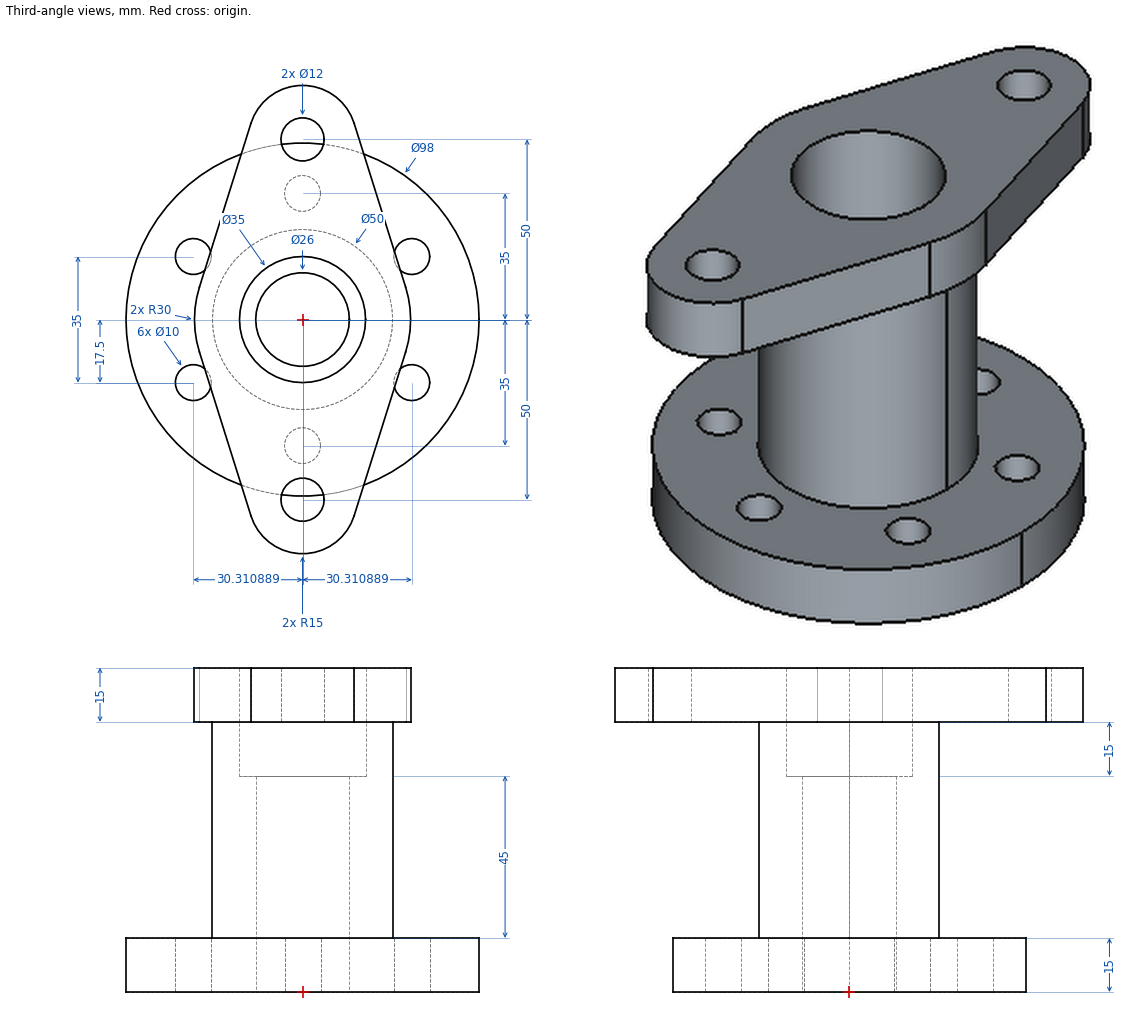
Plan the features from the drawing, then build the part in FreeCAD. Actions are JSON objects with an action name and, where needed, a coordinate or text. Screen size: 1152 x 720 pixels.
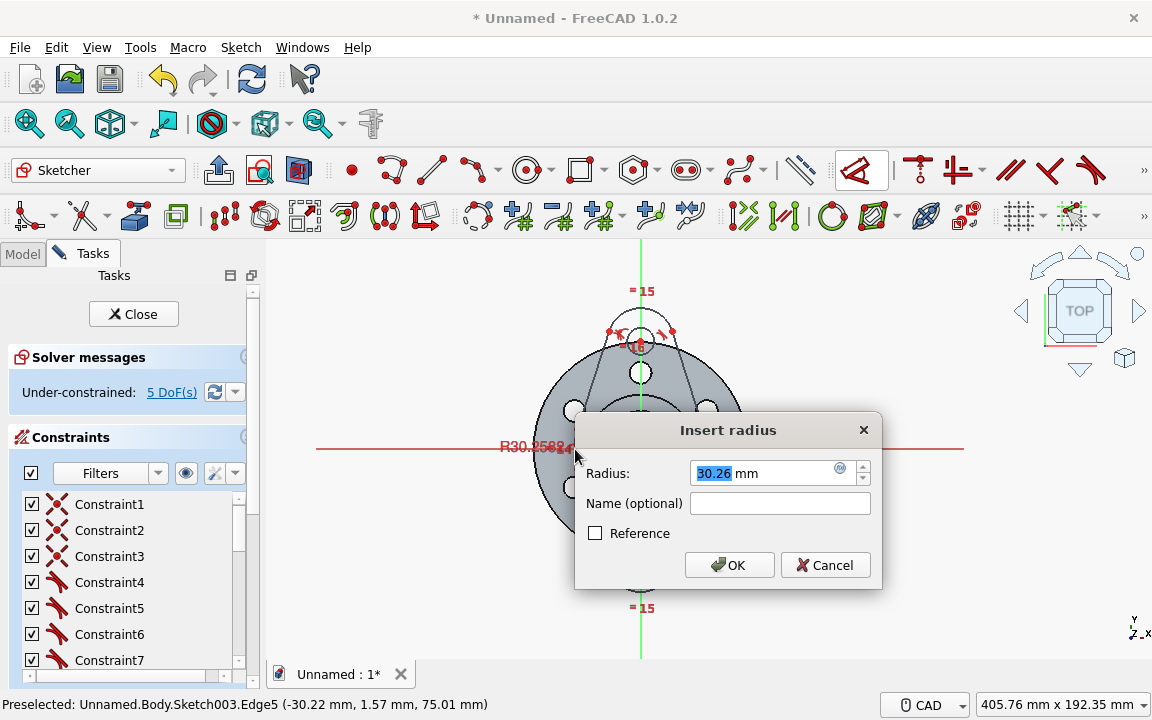
{"action": "type", "text": "30"}
{"action": "key", "text": "Return"}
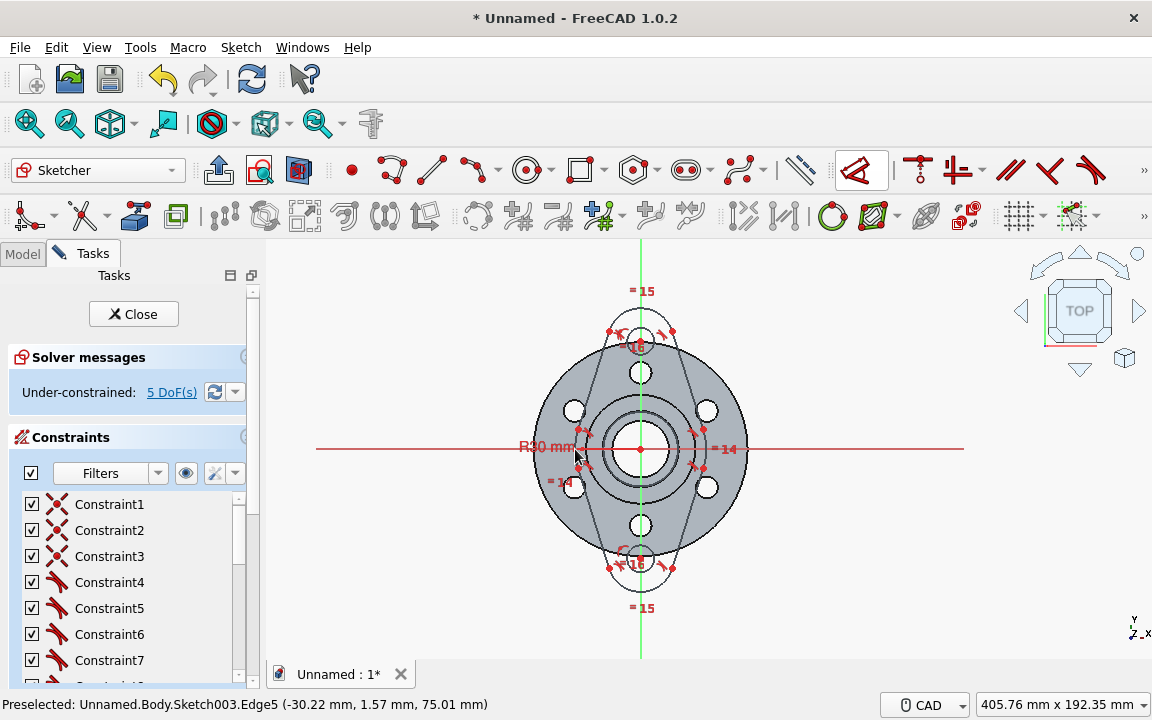
{"action": "left_click", "coordinate": [625, 588]}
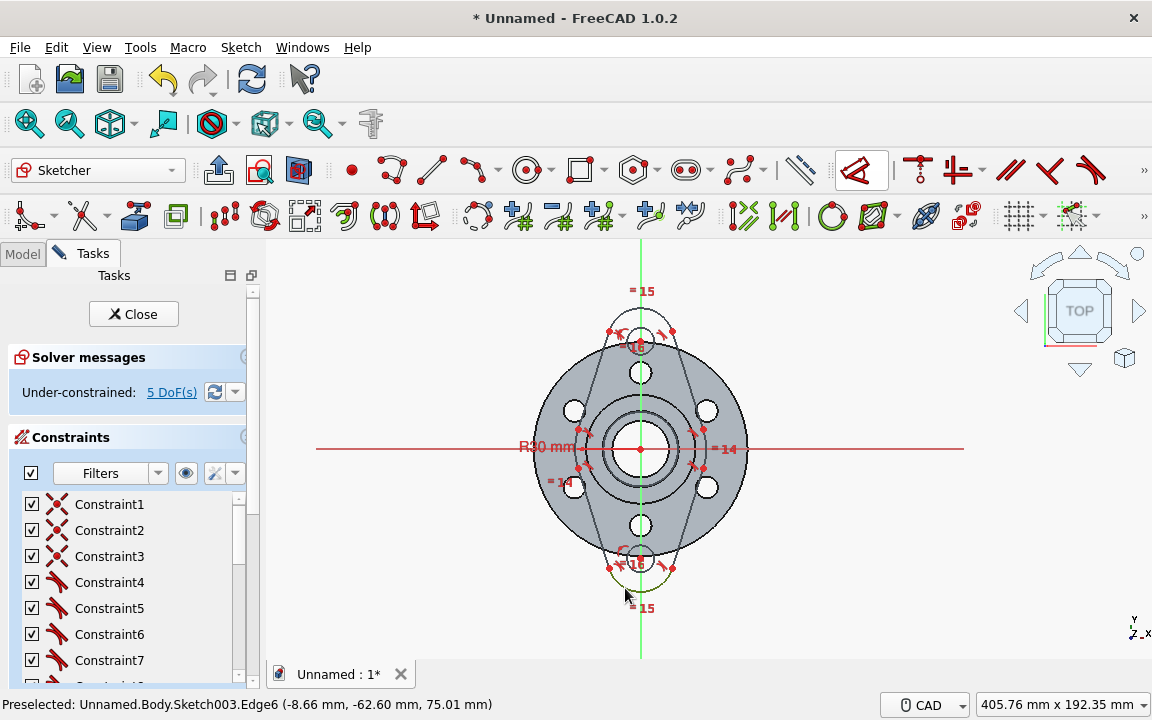
{"action": "key", "text": "k r"}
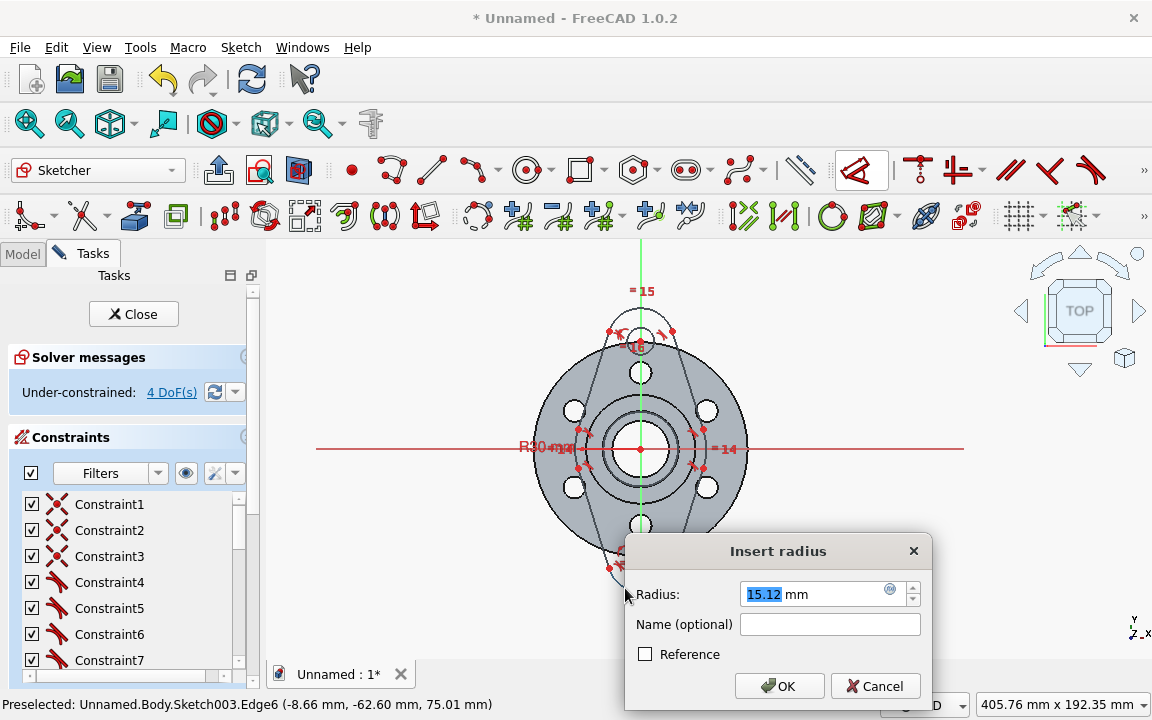
{"action": "type", "text": "15"}
{"action": "key", "text": "Return"}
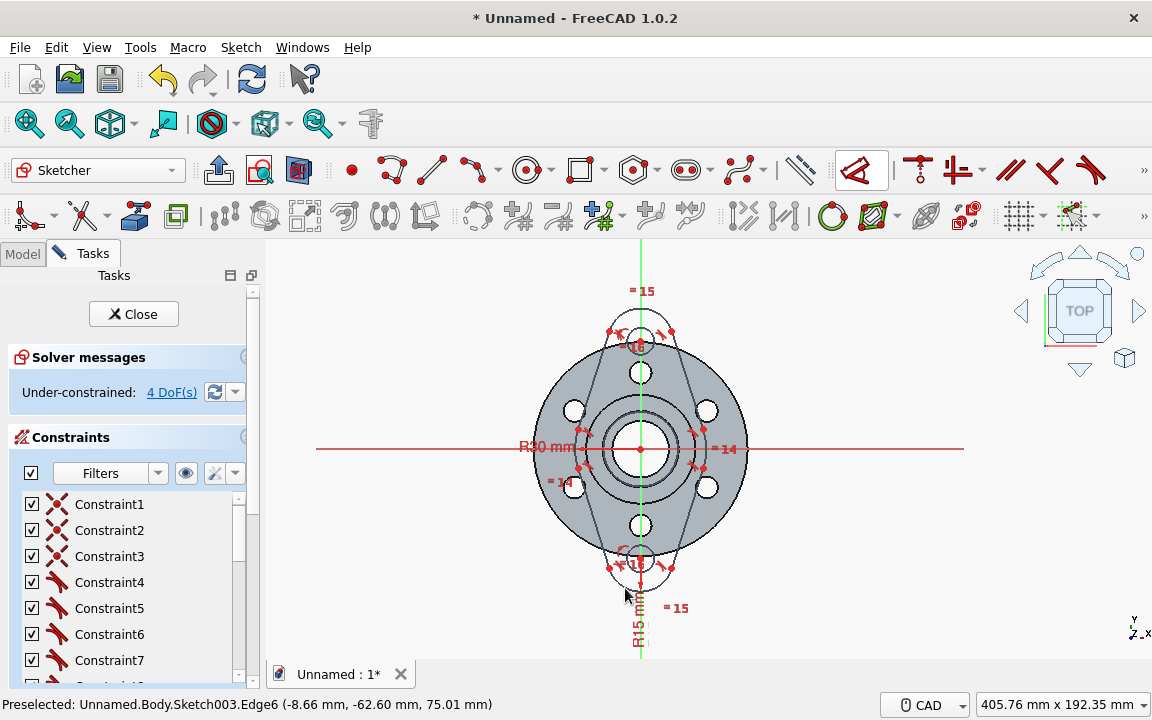
{"action": "scroll", "coordinate": [650, 332], "scroll_direction": "up", "scroll_amount": 3}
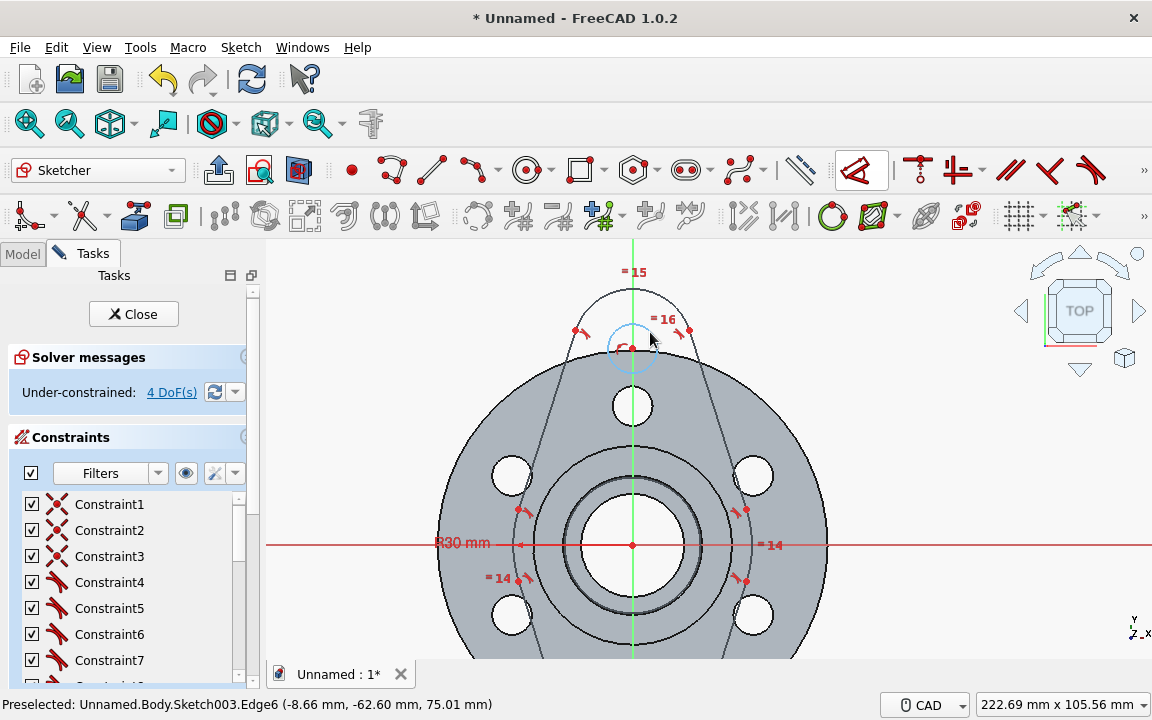
{"action": "left_click", "coordinate": [650, 331]}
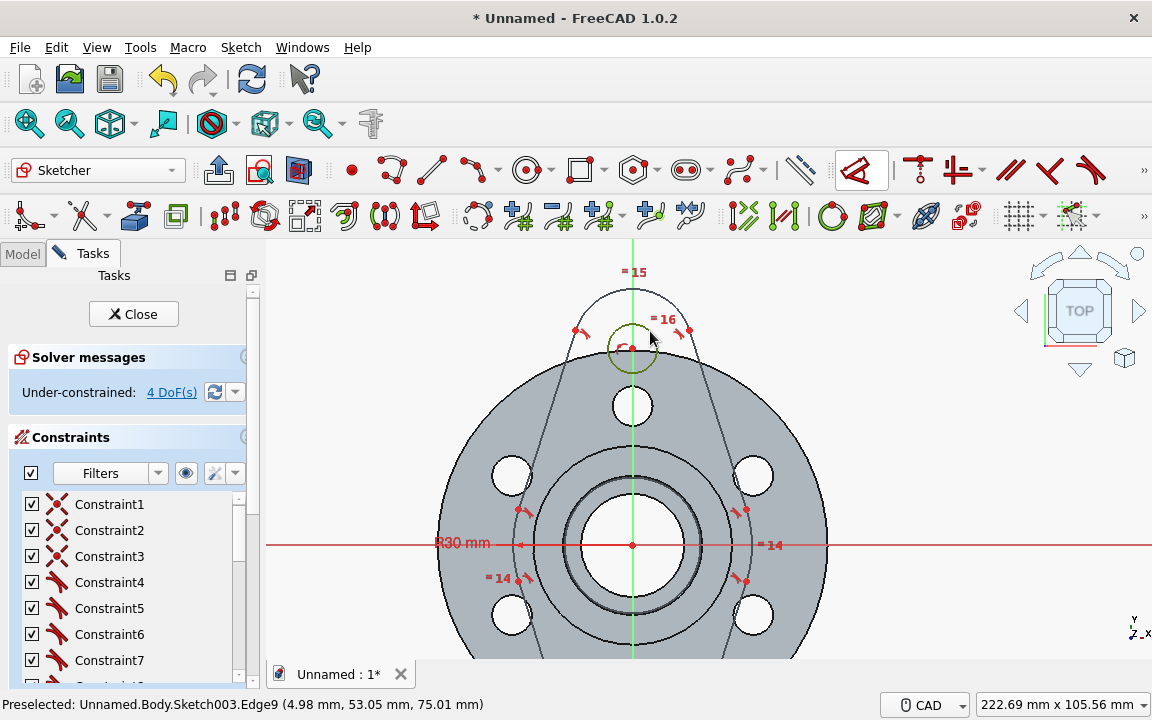
{"action": "left_click", "coordinate": [882, 170]}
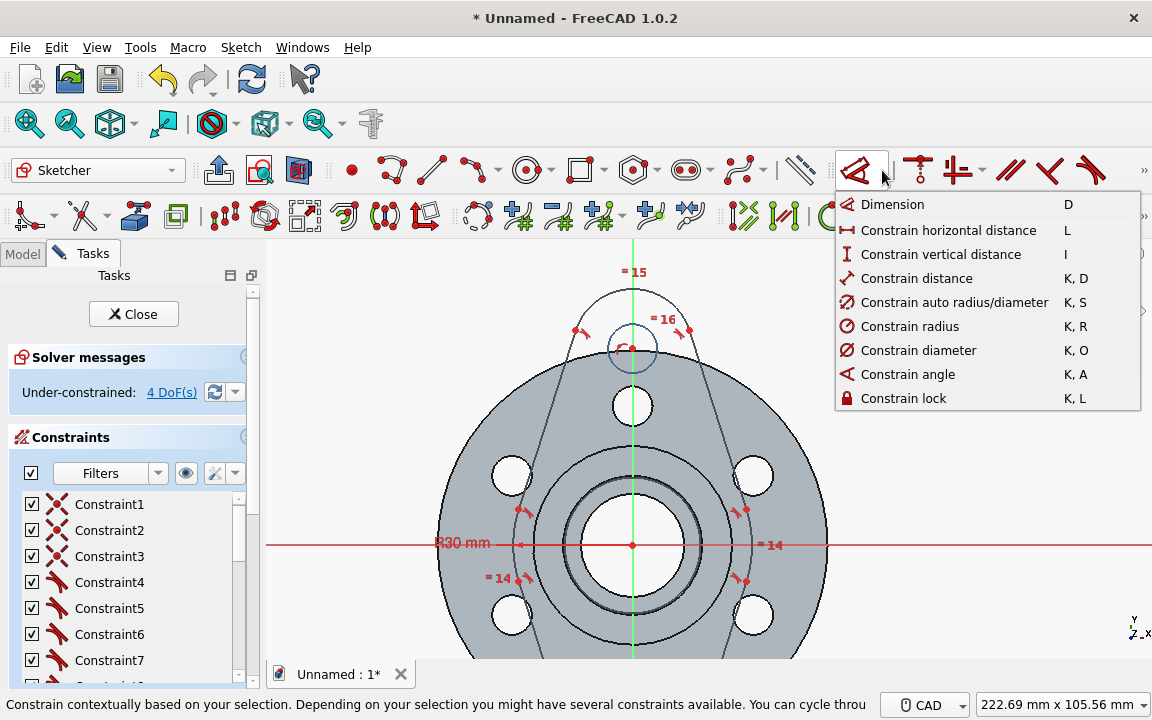
{"action": "left_click", "coordinate": [988, 350]}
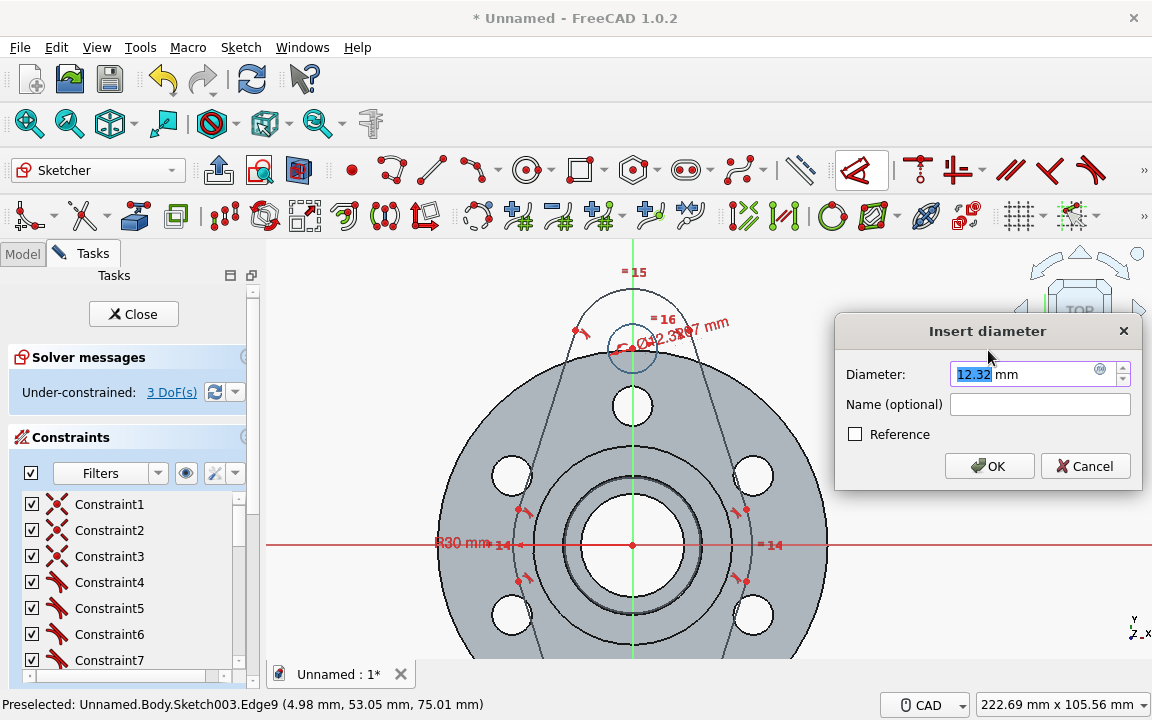
{"action": "type", "text": "12"}
{"action": "key", "text": "Return"}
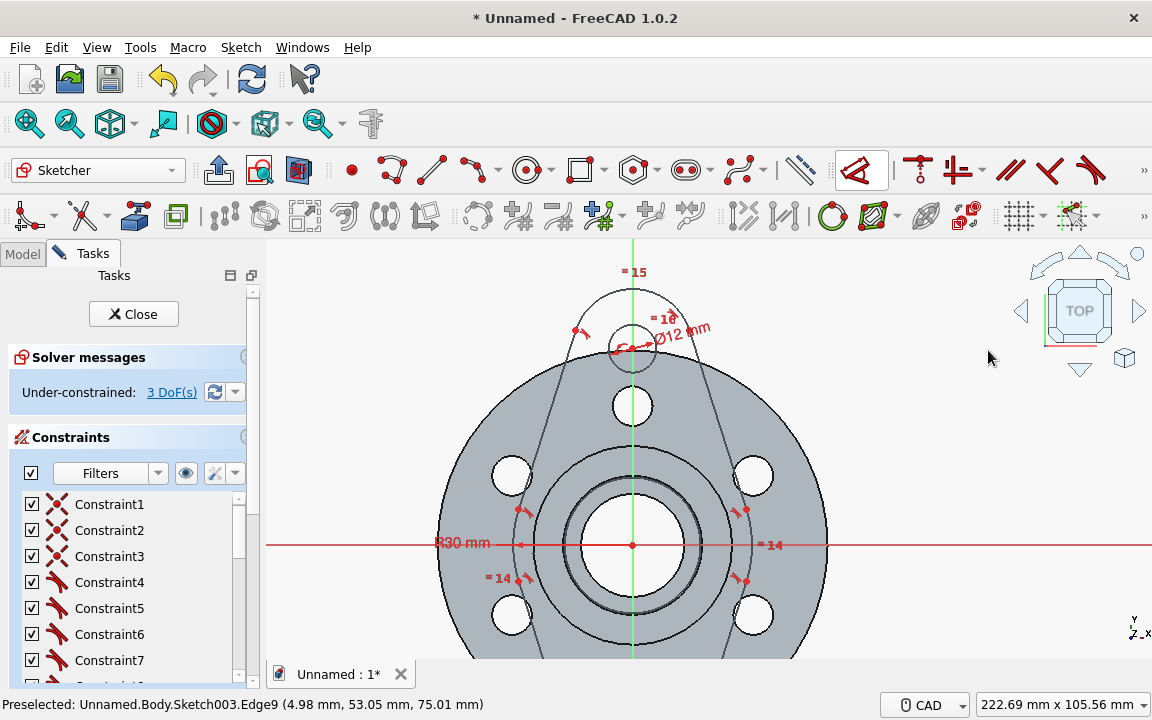
{"action": "left_click", "coordinate": [681, 497]}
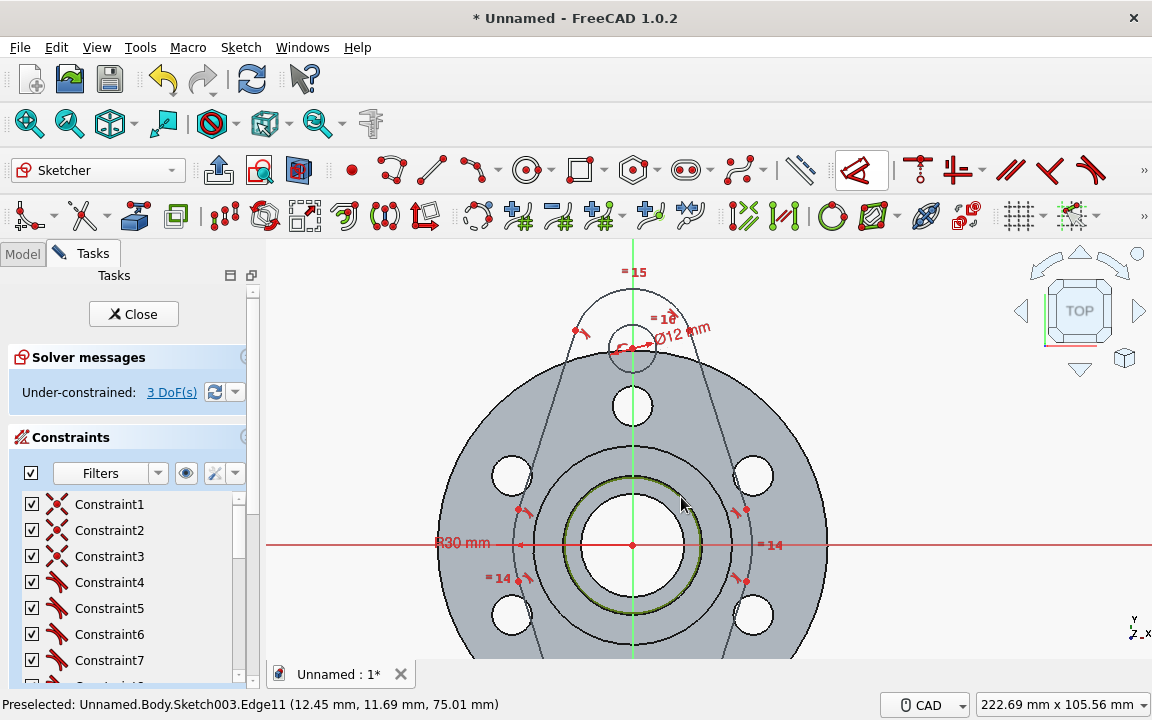
{"action": "key", "text": "k o"}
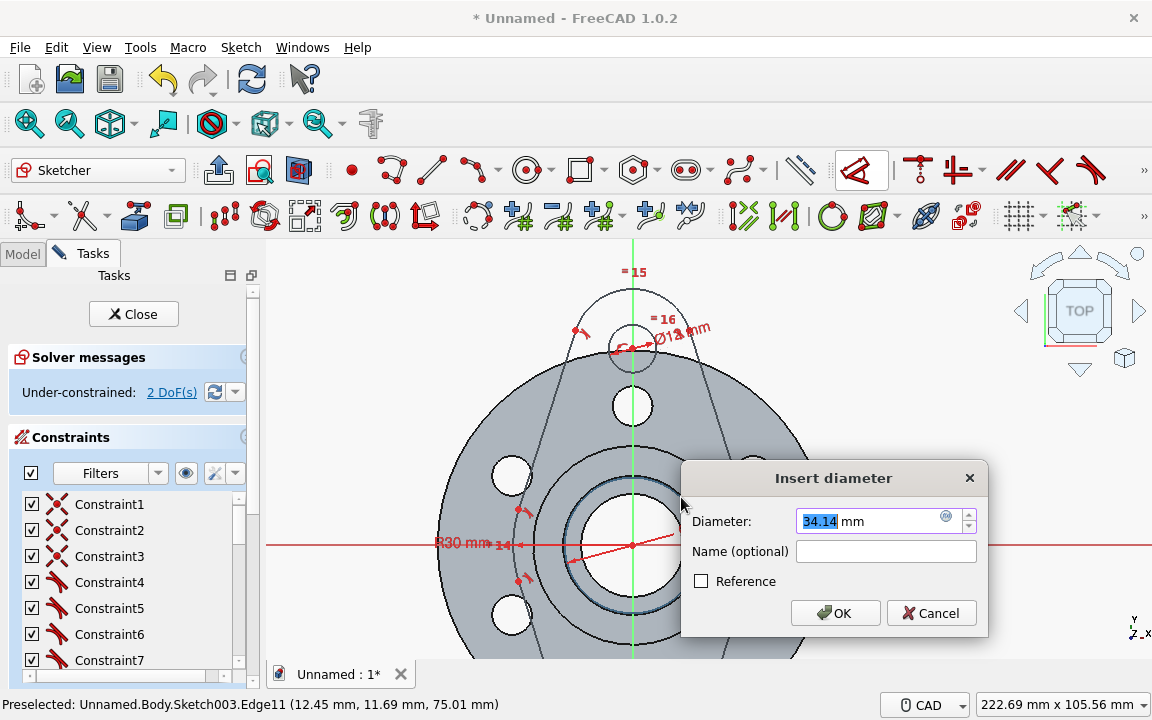
{"action": "type", "text": "35"}
{"action": "key", "text": "Return"}